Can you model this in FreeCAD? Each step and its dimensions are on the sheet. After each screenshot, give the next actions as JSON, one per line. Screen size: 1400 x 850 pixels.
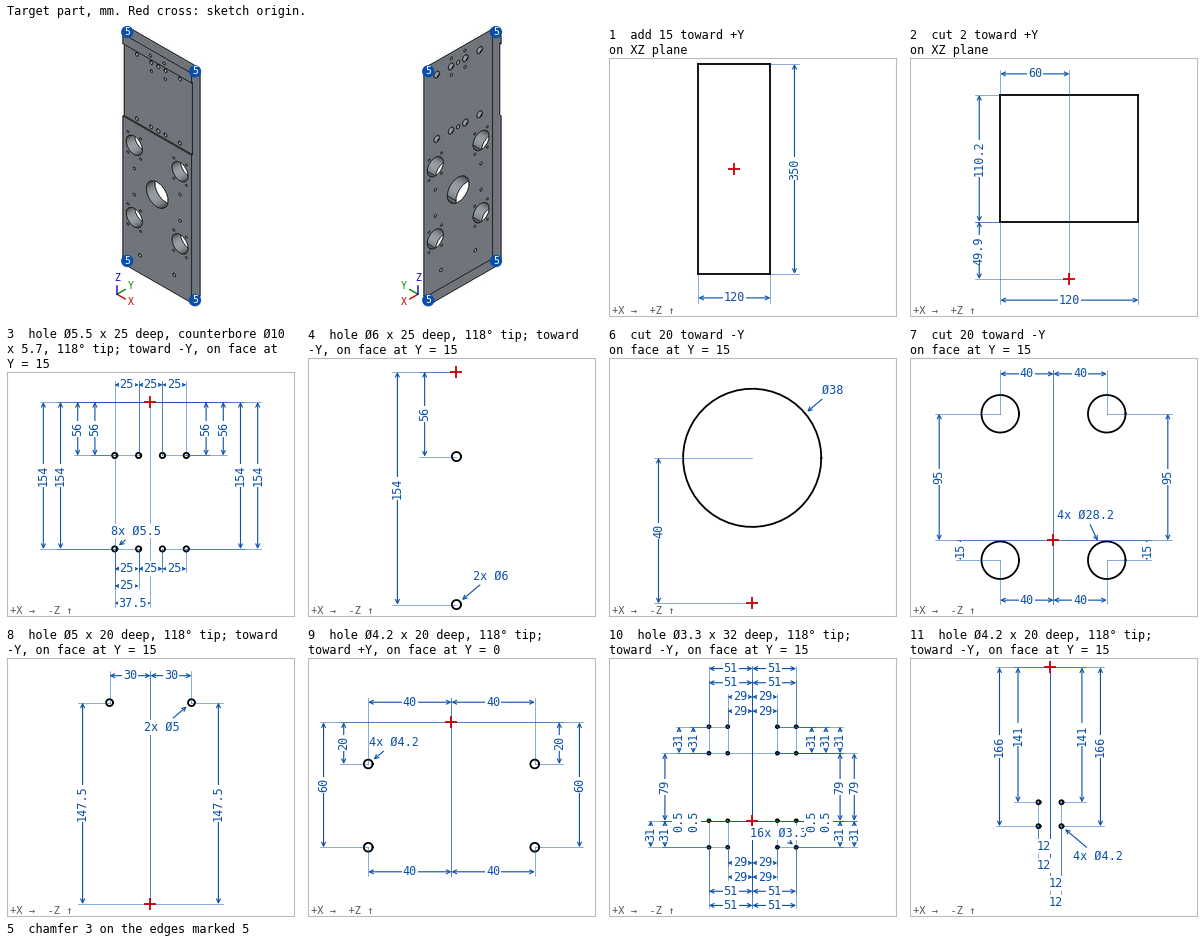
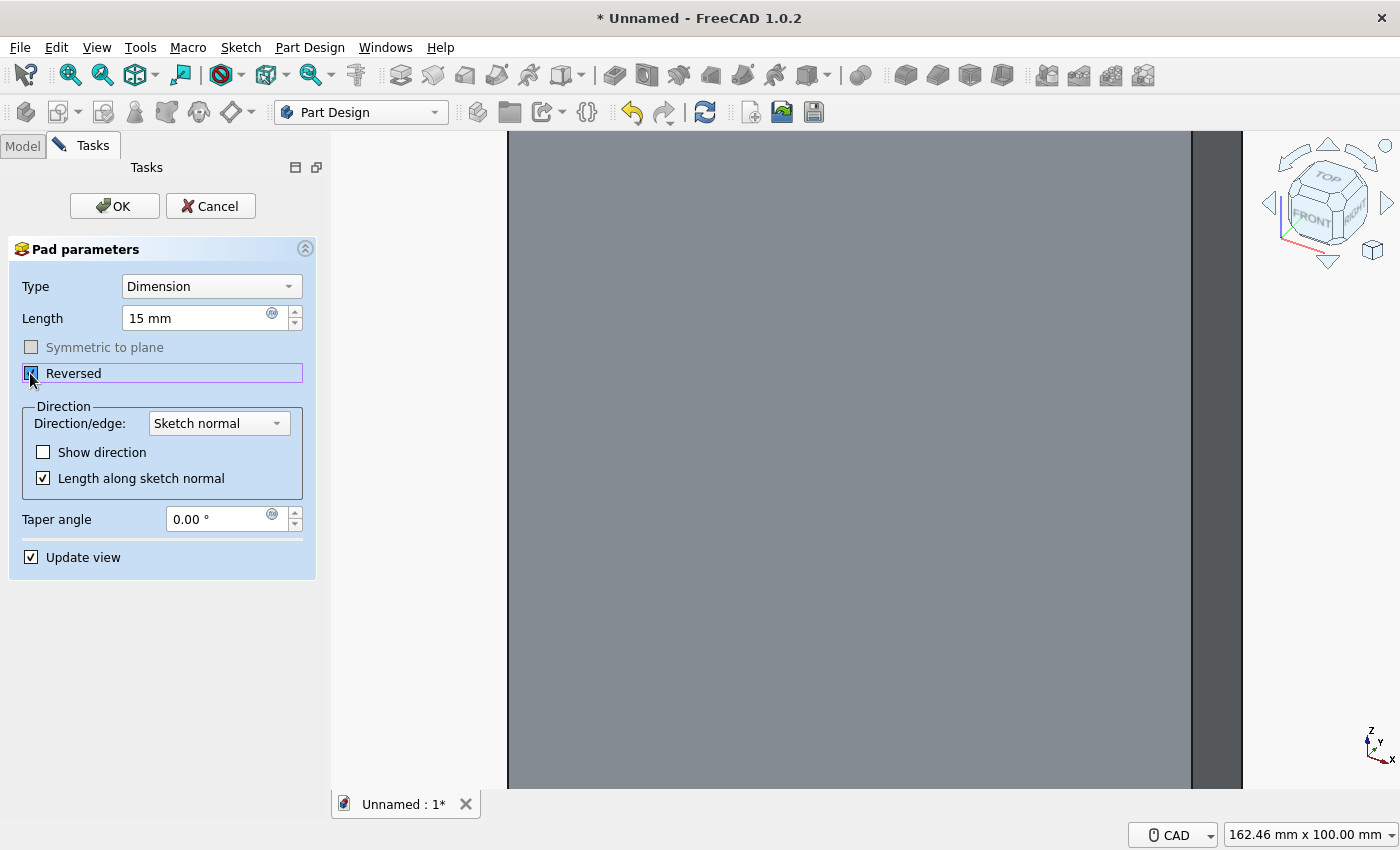
{"action": "left_click", "coordinate": [115, 206]}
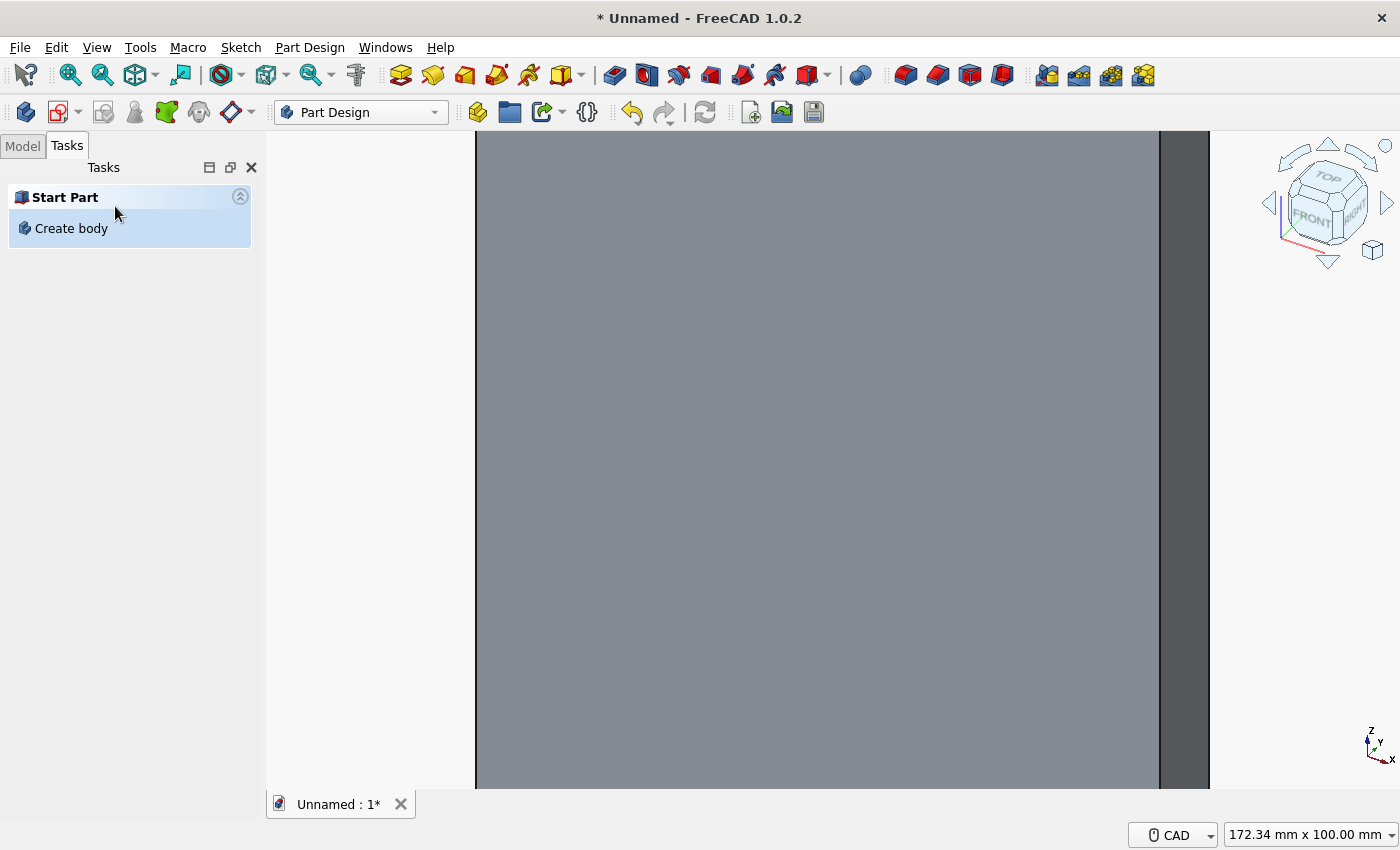
{"action": "left_click", "coordinate": [72, 76]}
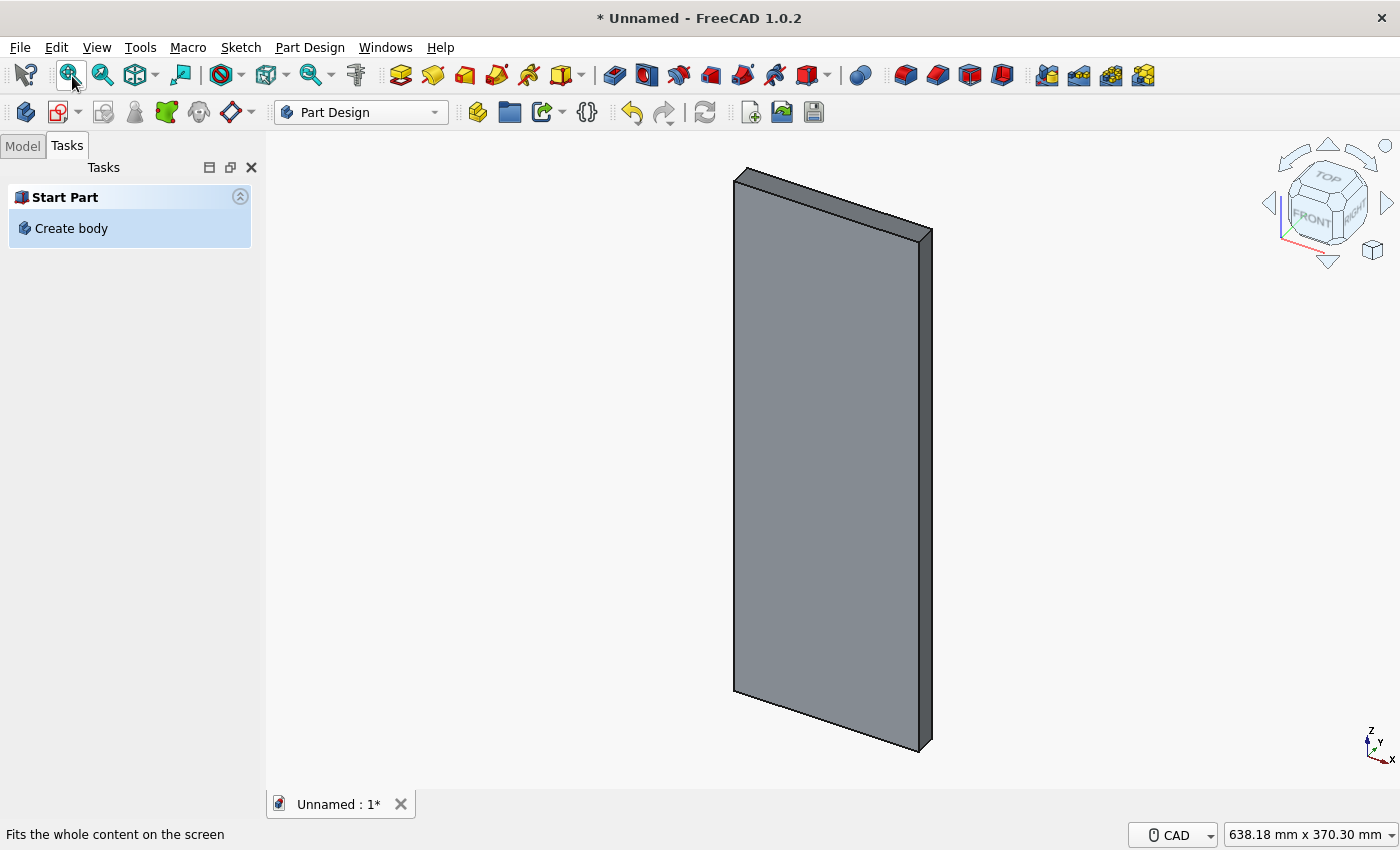
{"action": "left_click", "coordinate": [58, 112]}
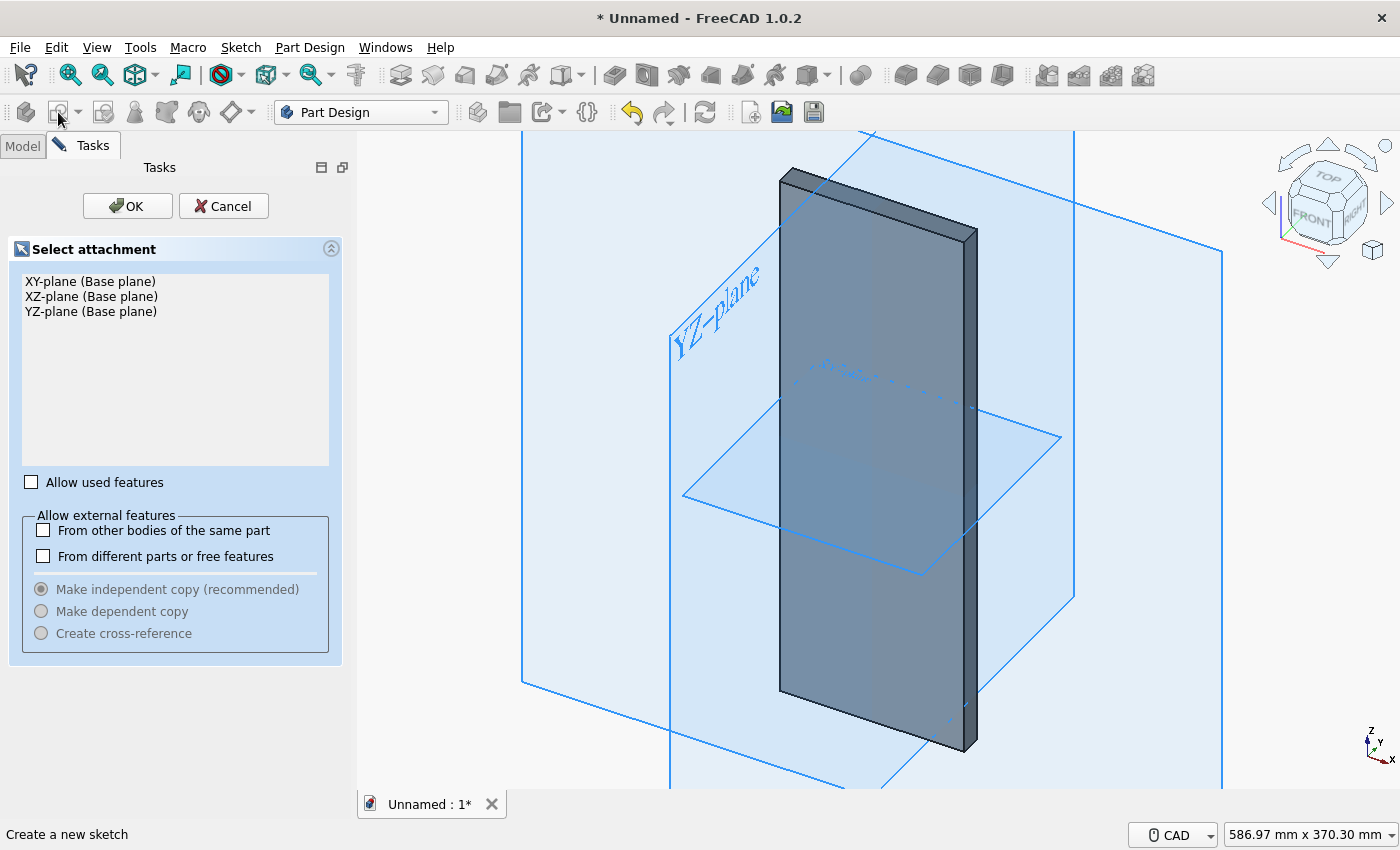
{"action": "left_click", "coordinate": [82, 296]}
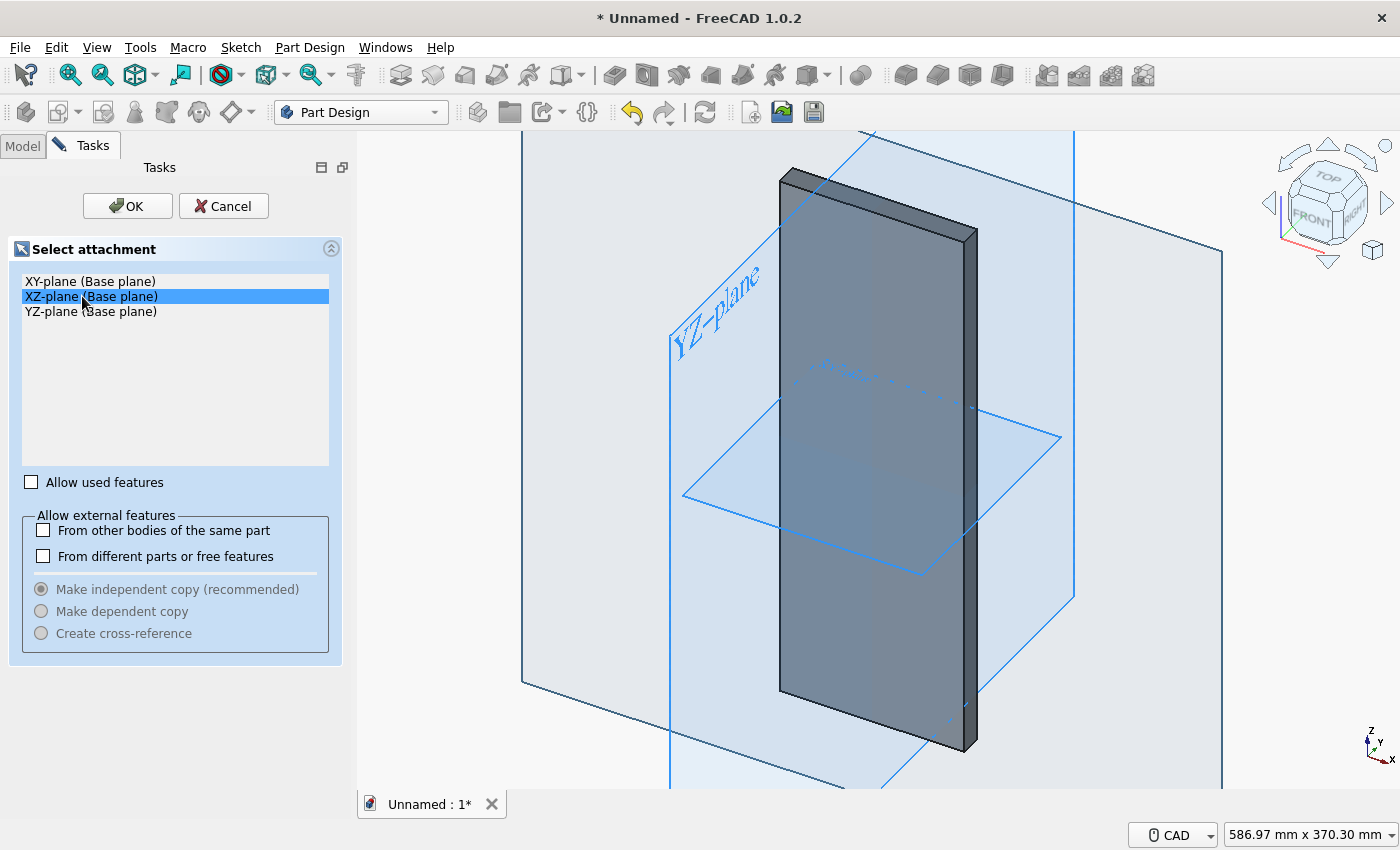
{"action": "left_click", "coordinate": [128, 206]}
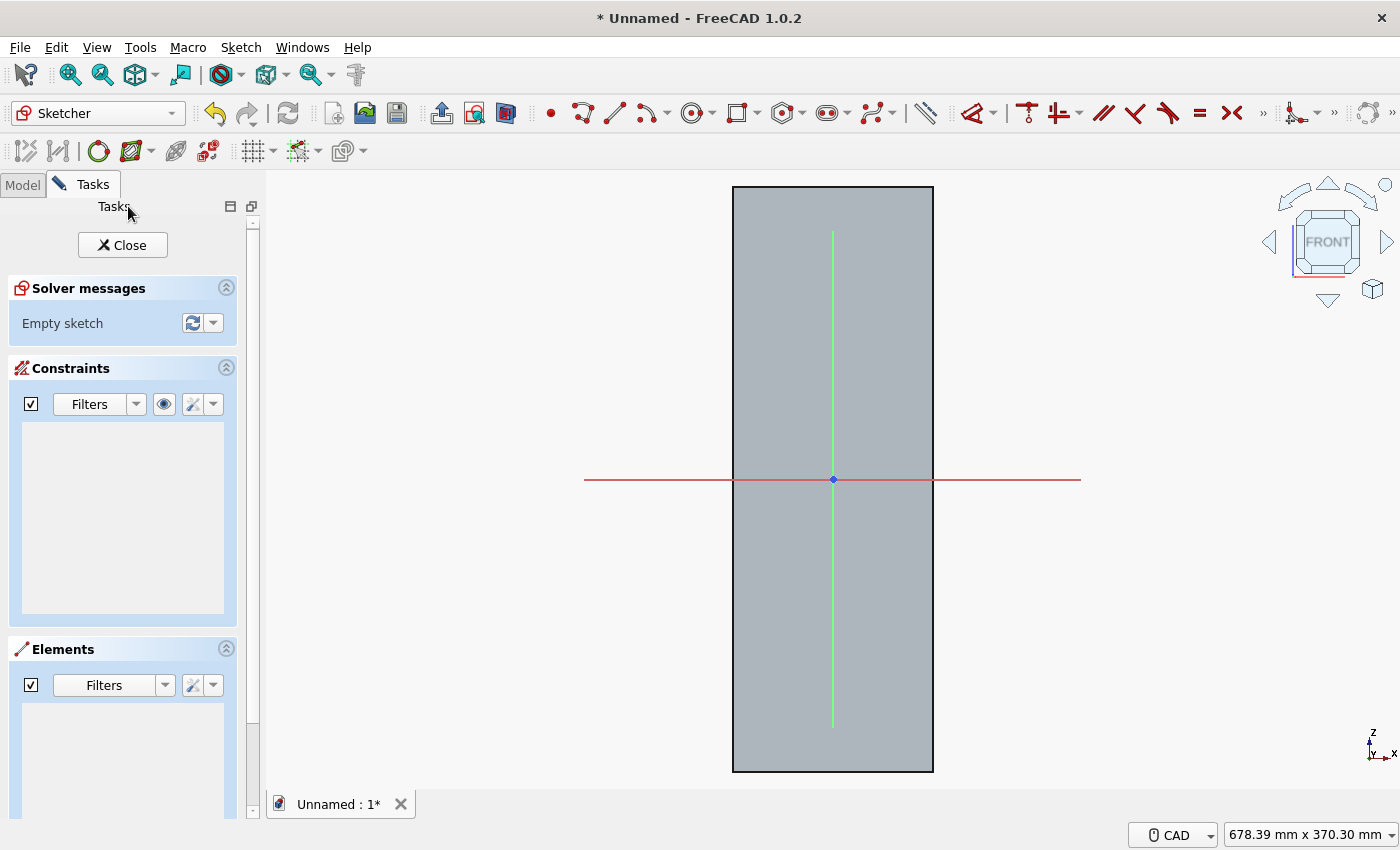
{"action": "scroll", "coordinate": [455, 761], "scroll_direction": "down", "scroll_amount": 1}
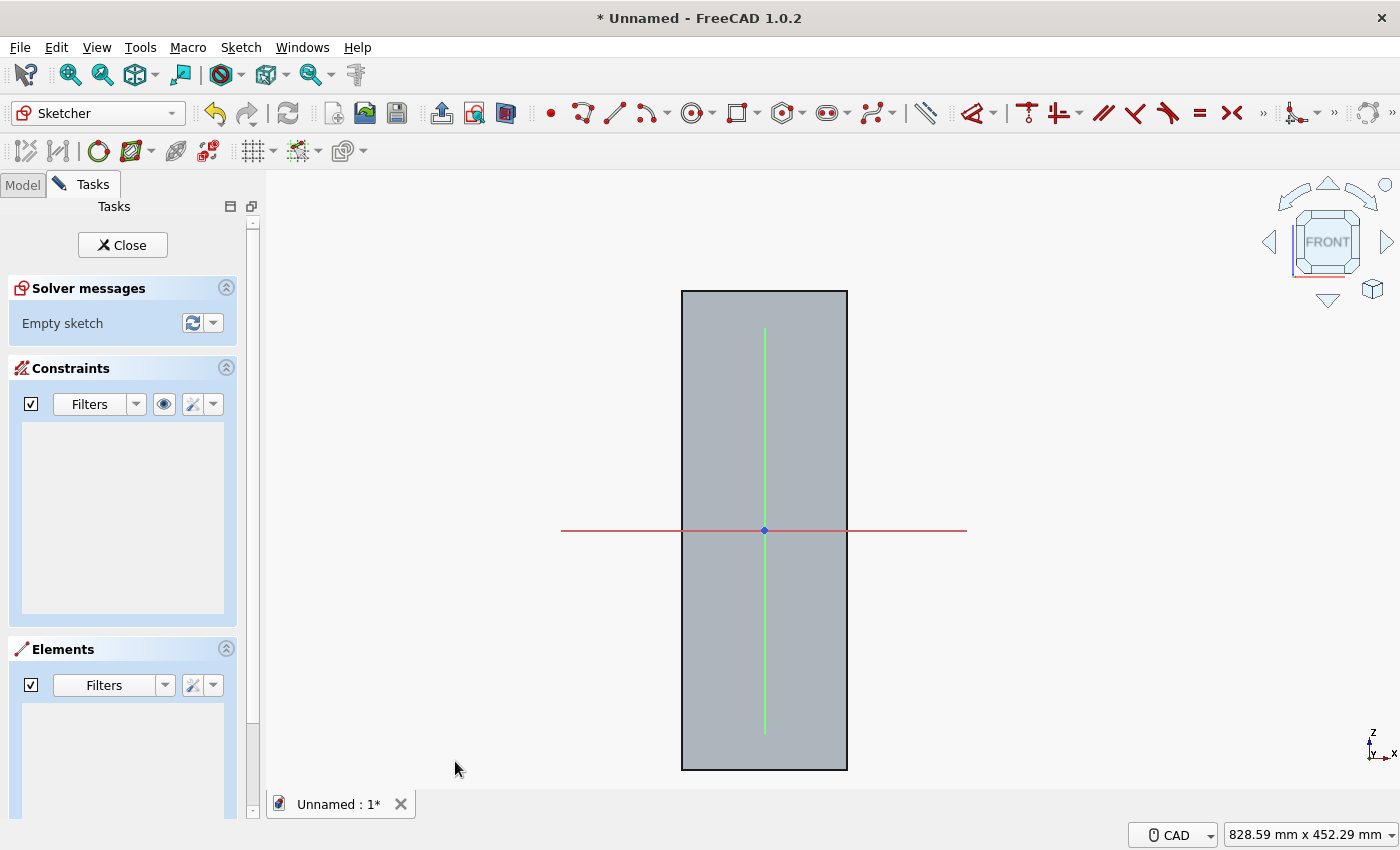
{"action": "scroll", "coordinate": [765, 350], "scroll_direction": "up", "scroll_amount": 3}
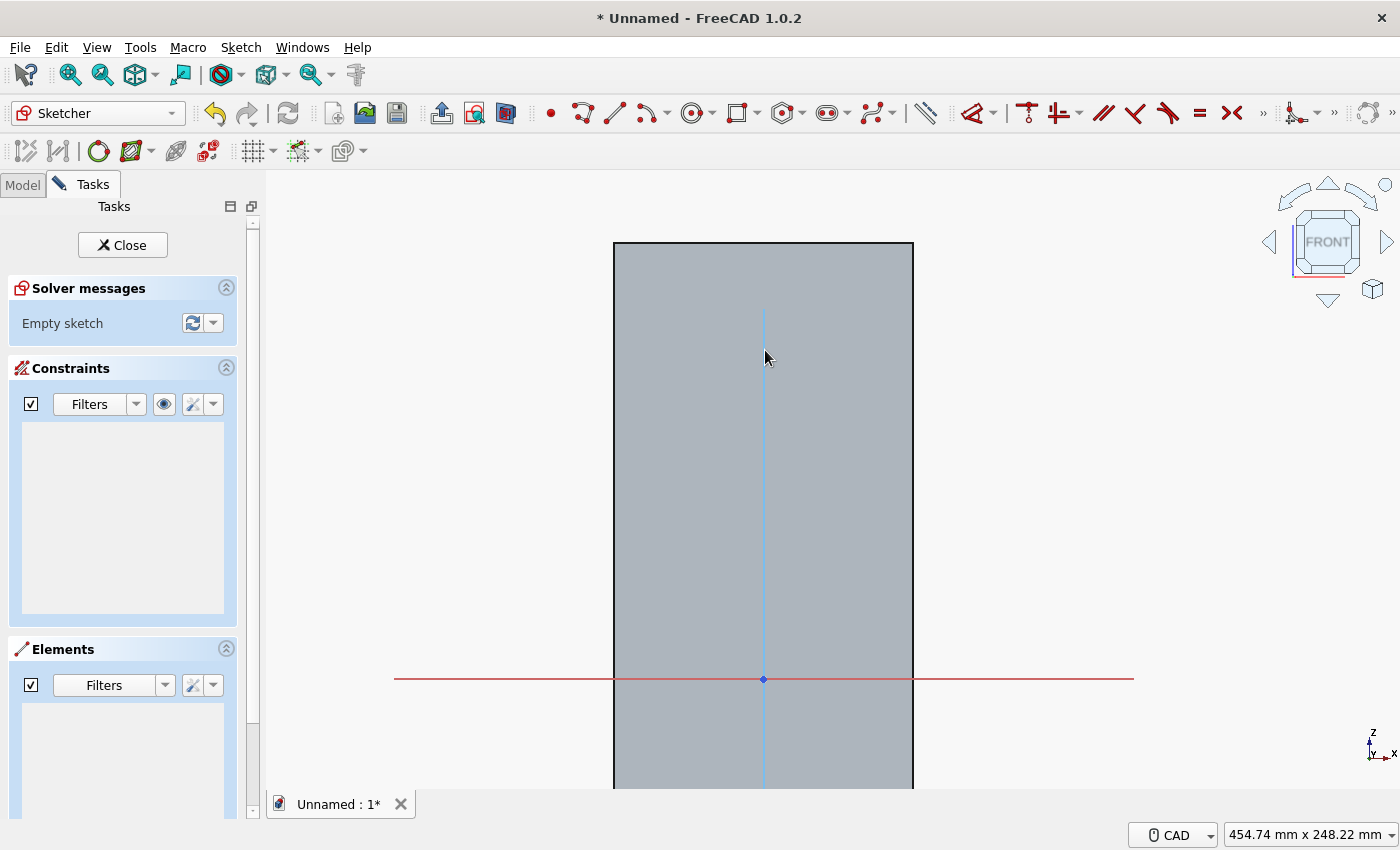
{"action": "left_click", "coordinate": [738, 114]}